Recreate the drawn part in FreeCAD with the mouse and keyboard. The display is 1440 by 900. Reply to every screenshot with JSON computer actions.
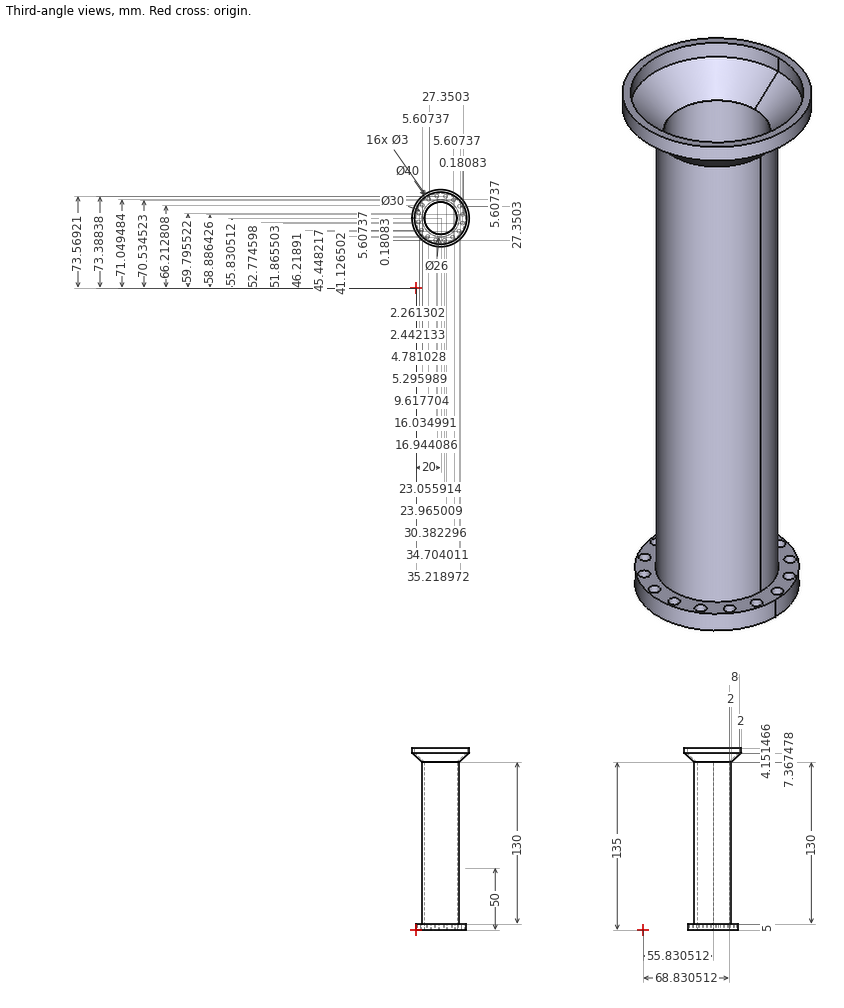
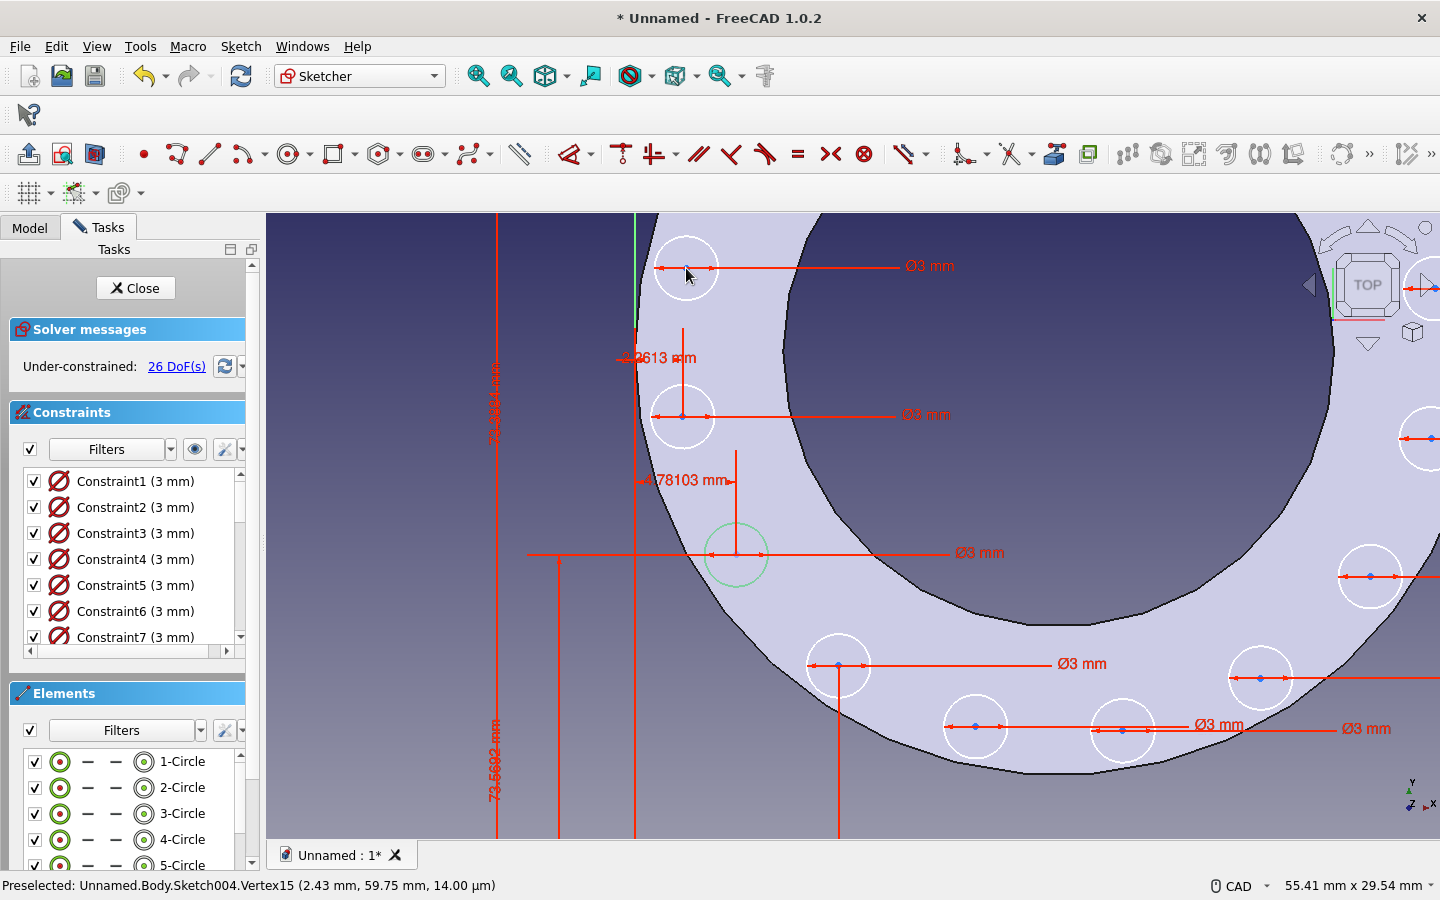
{"action": "left_click", "coordinate": [686, 268]}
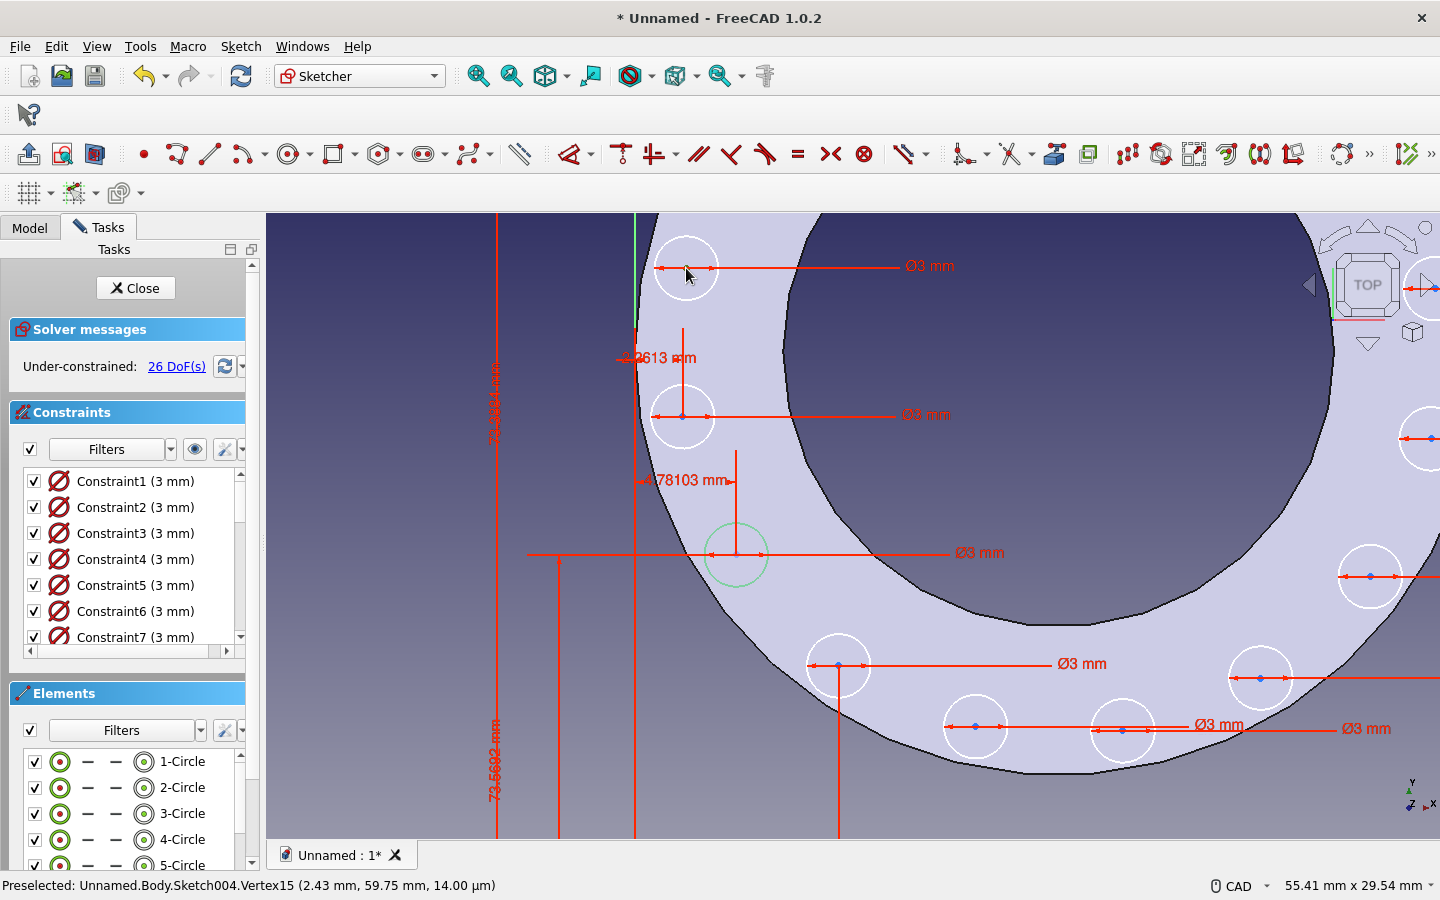
{"action": "key", "text": "l"}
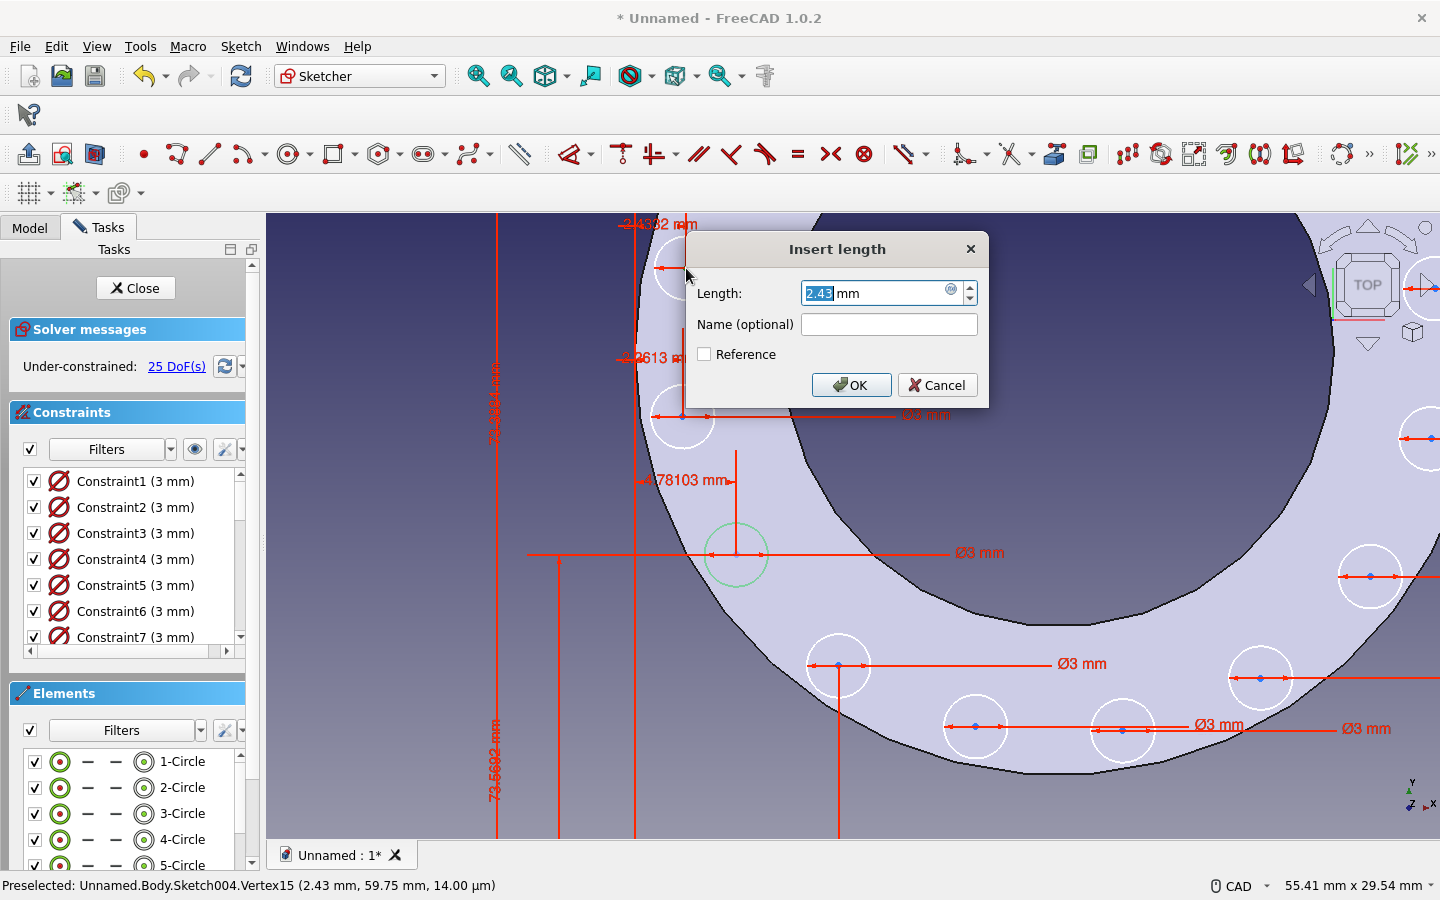
{"action": "type", "text": "2.442133"}
{"action": "key", "text": "Return"}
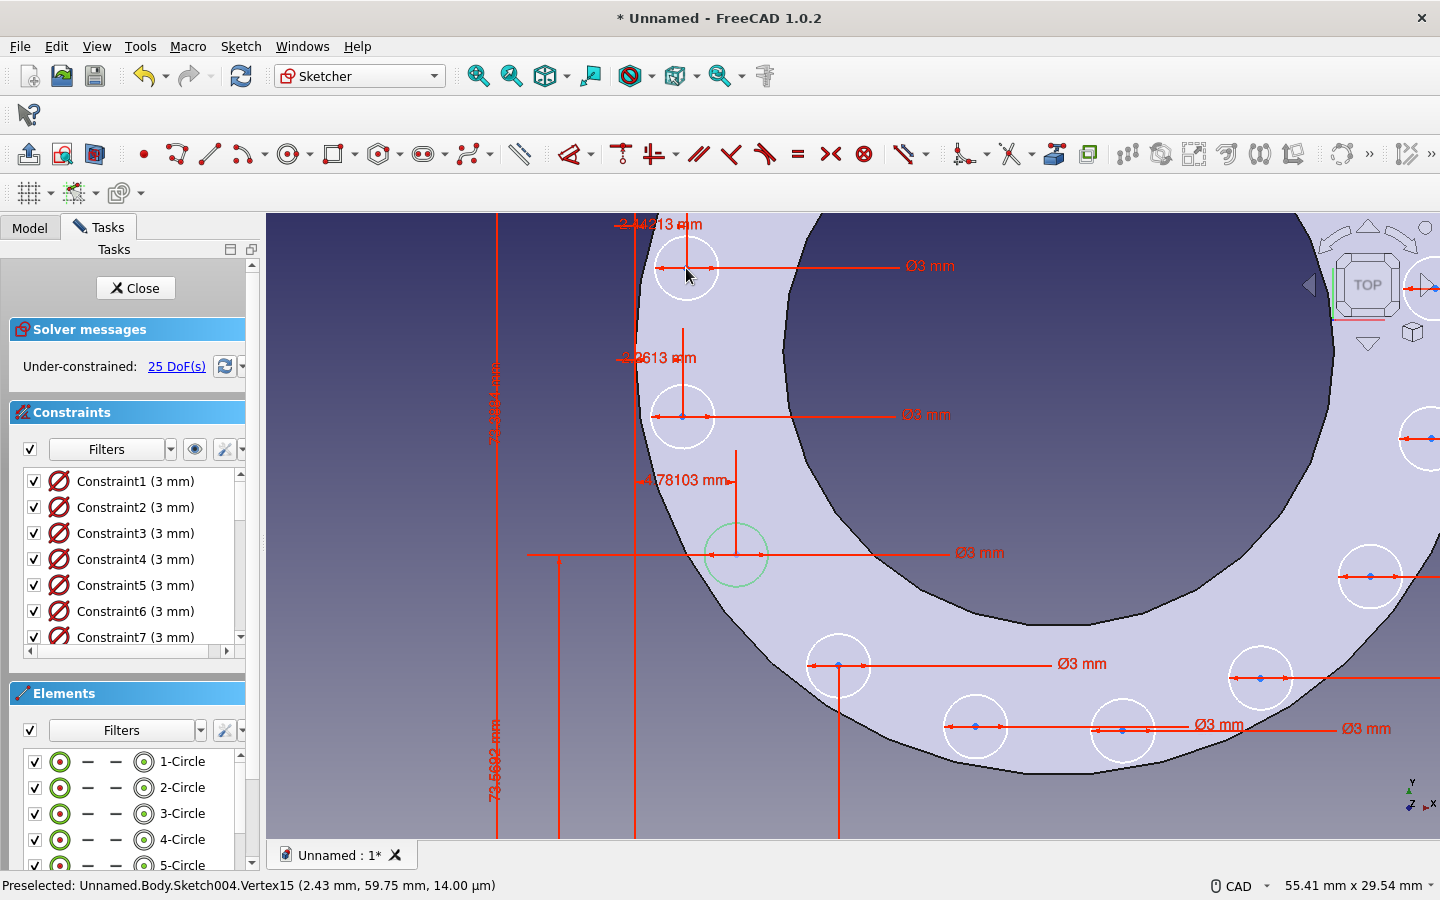
{"action": "scroll", "coordinate": [697, 456], "scroll_direction": "down", "scroll_amount": 7}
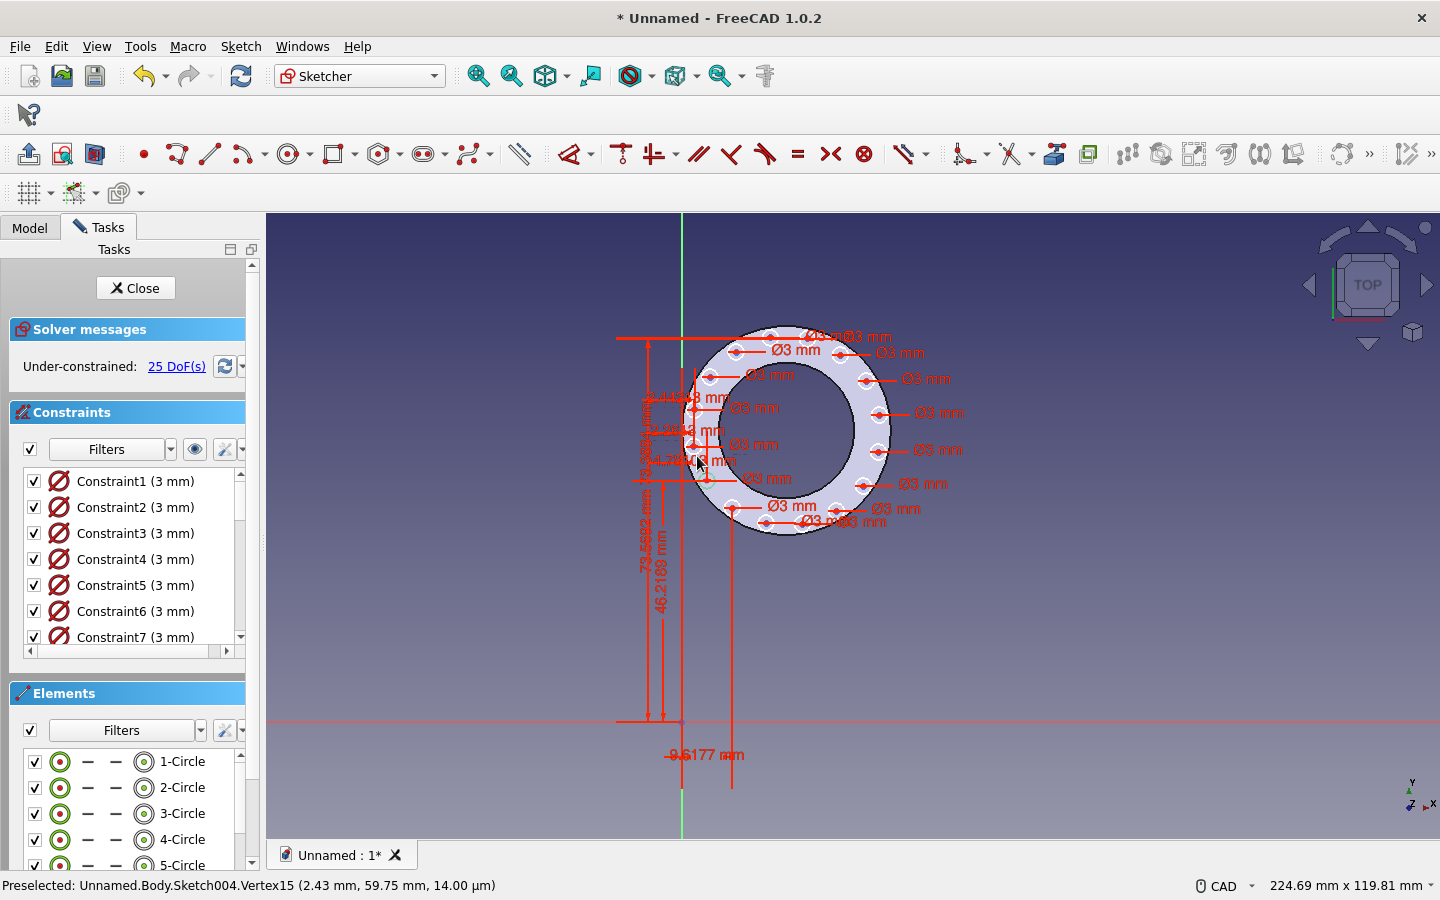
{"action": "scroll", "coordinate": [710, 377], "scroll_direction": "up", "scroll_amount": 2}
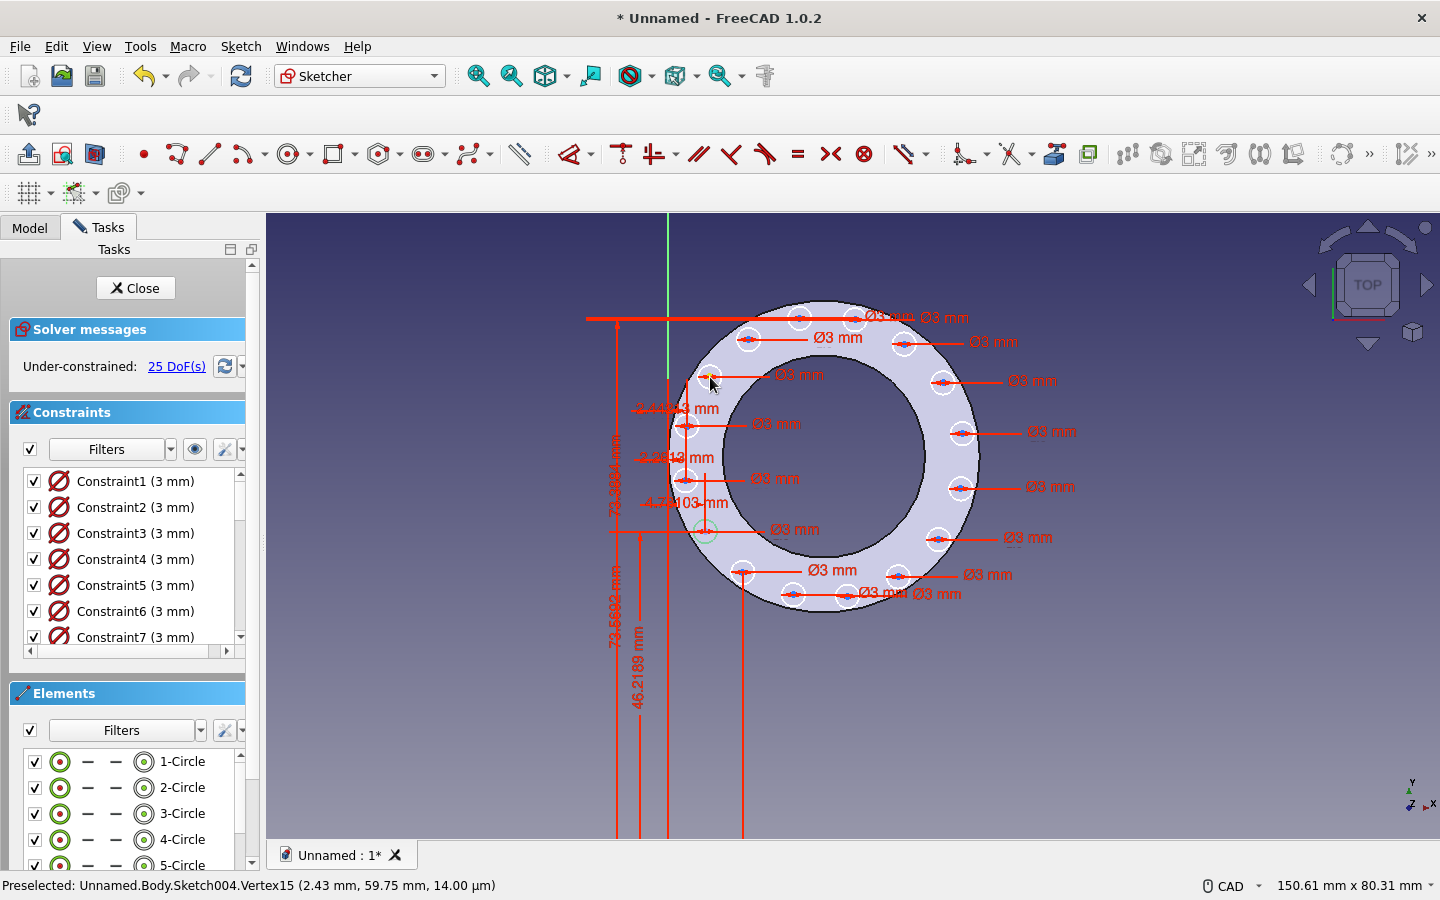
{"action": "left_click", "coordinate": [710, 377]}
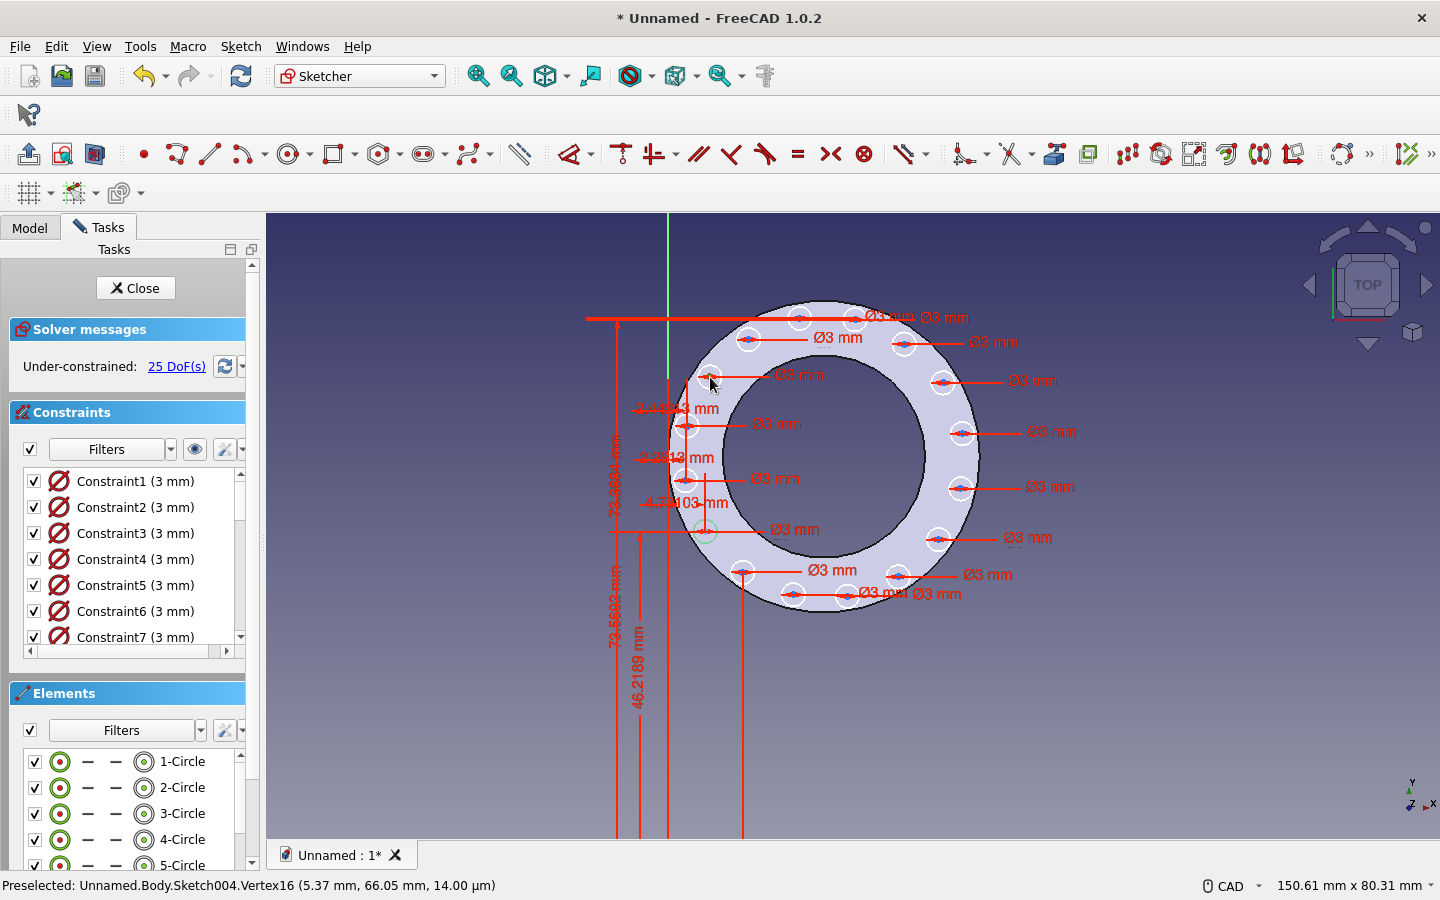
{"action": "left_click", "coordinate": [590, 154]}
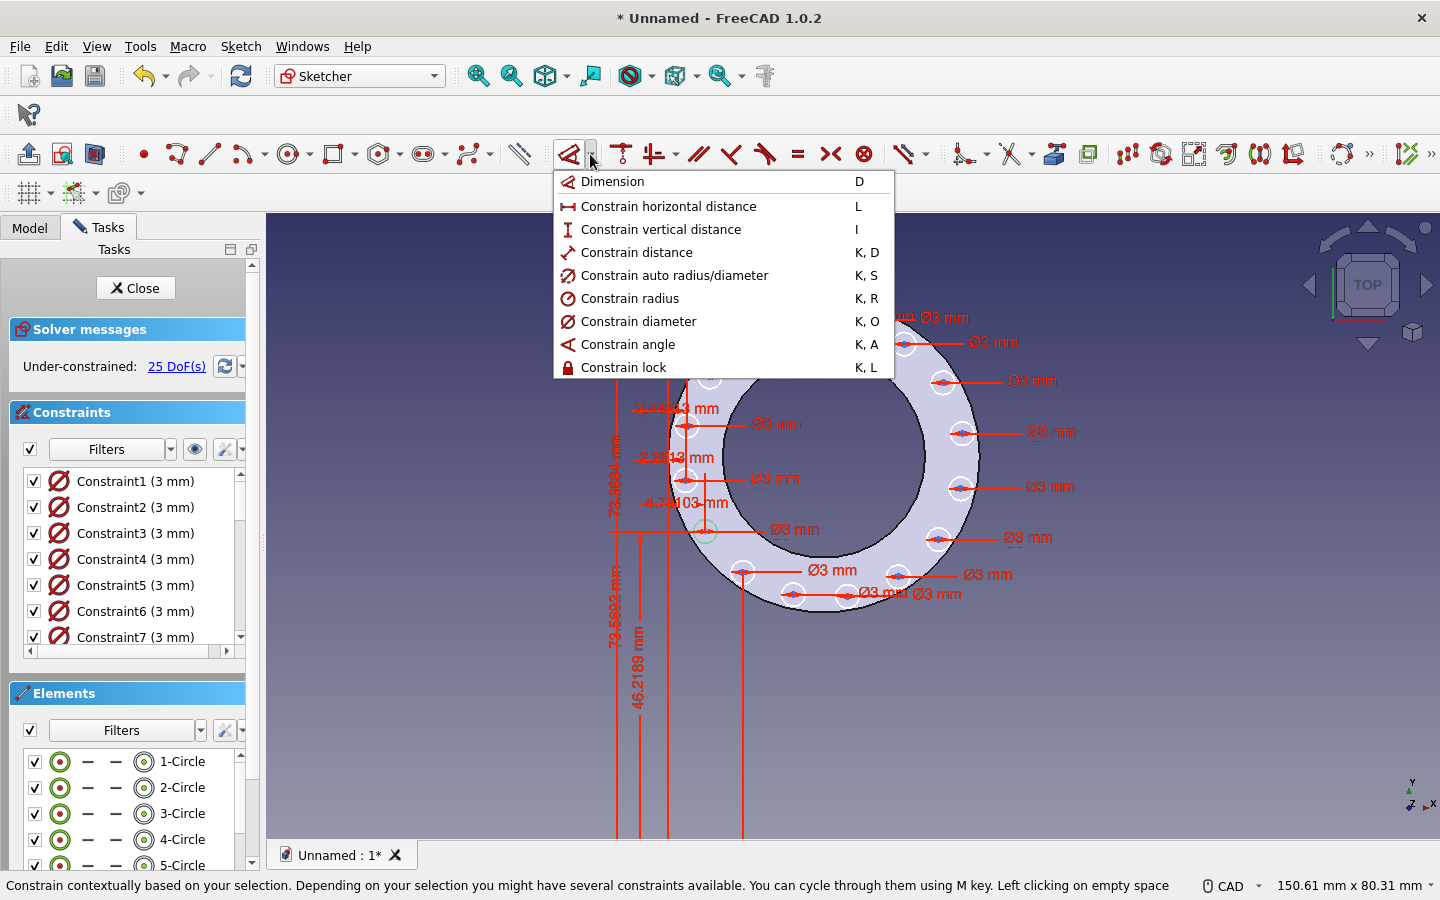
{"action": "left_click", "coordinate": [724, 206]}